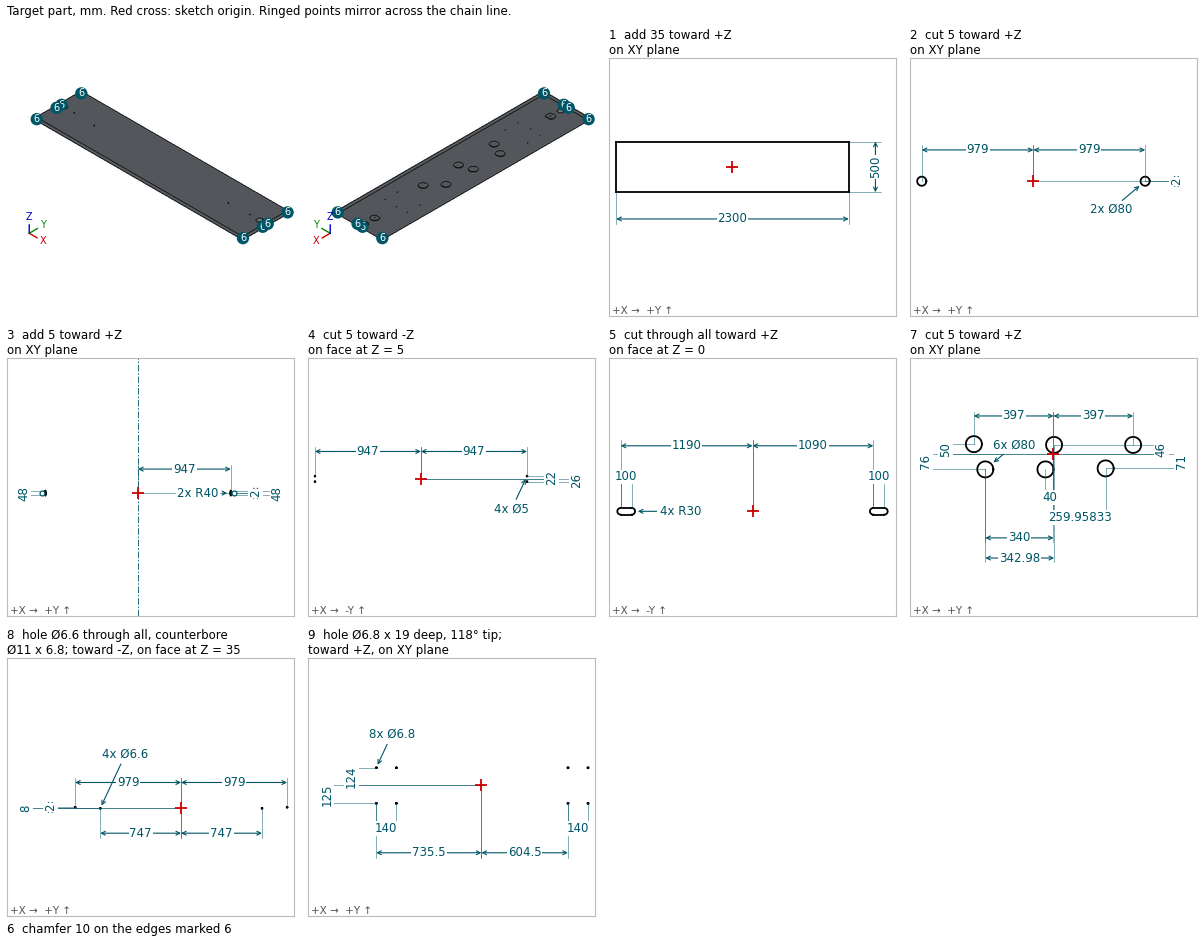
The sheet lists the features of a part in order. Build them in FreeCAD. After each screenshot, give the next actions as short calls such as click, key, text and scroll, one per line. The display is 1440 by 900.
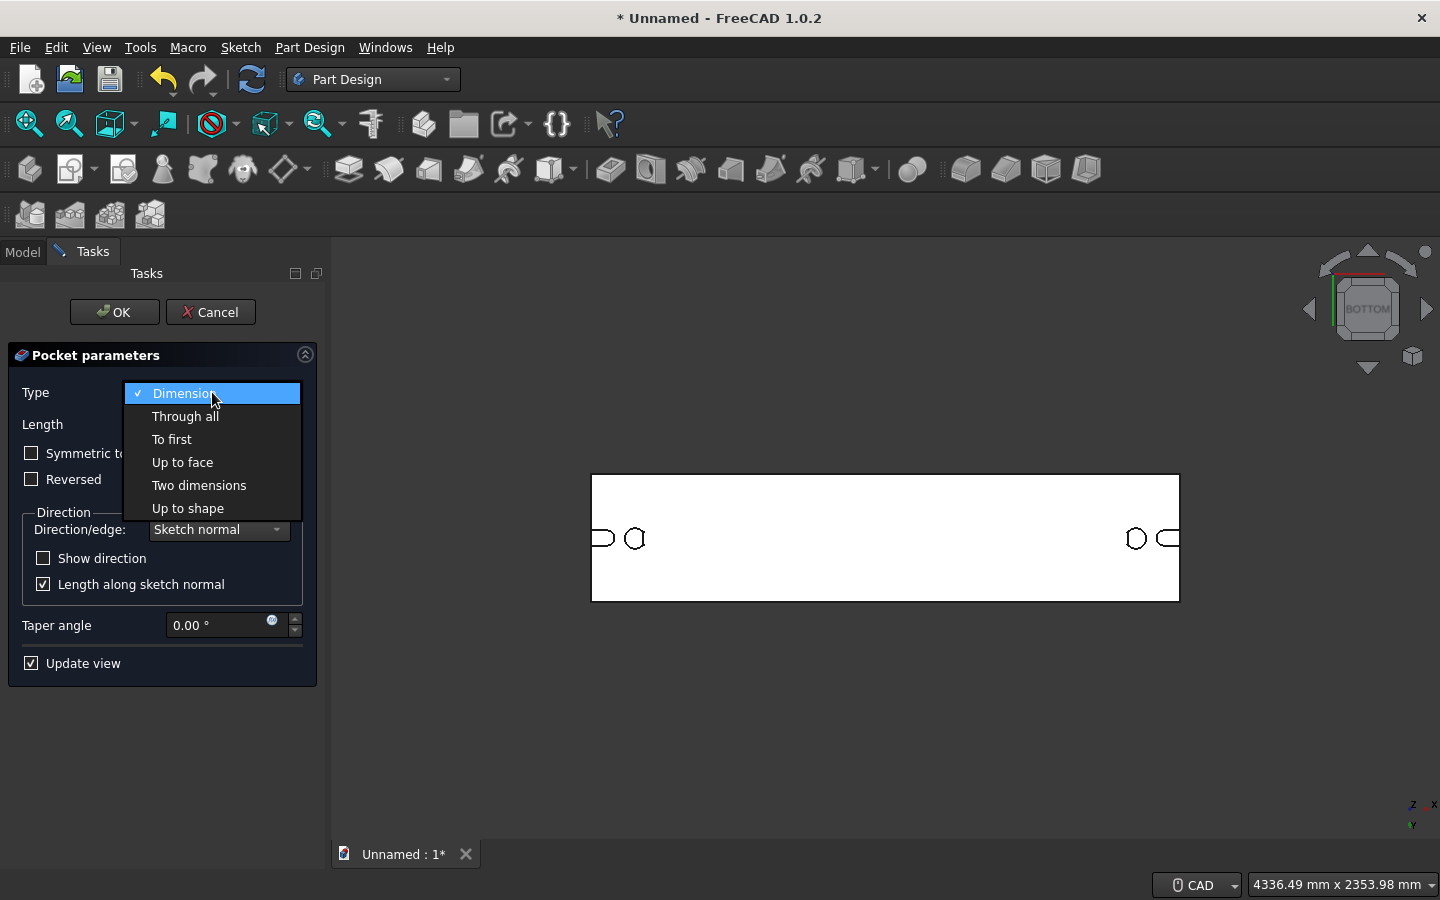
click(212, 416)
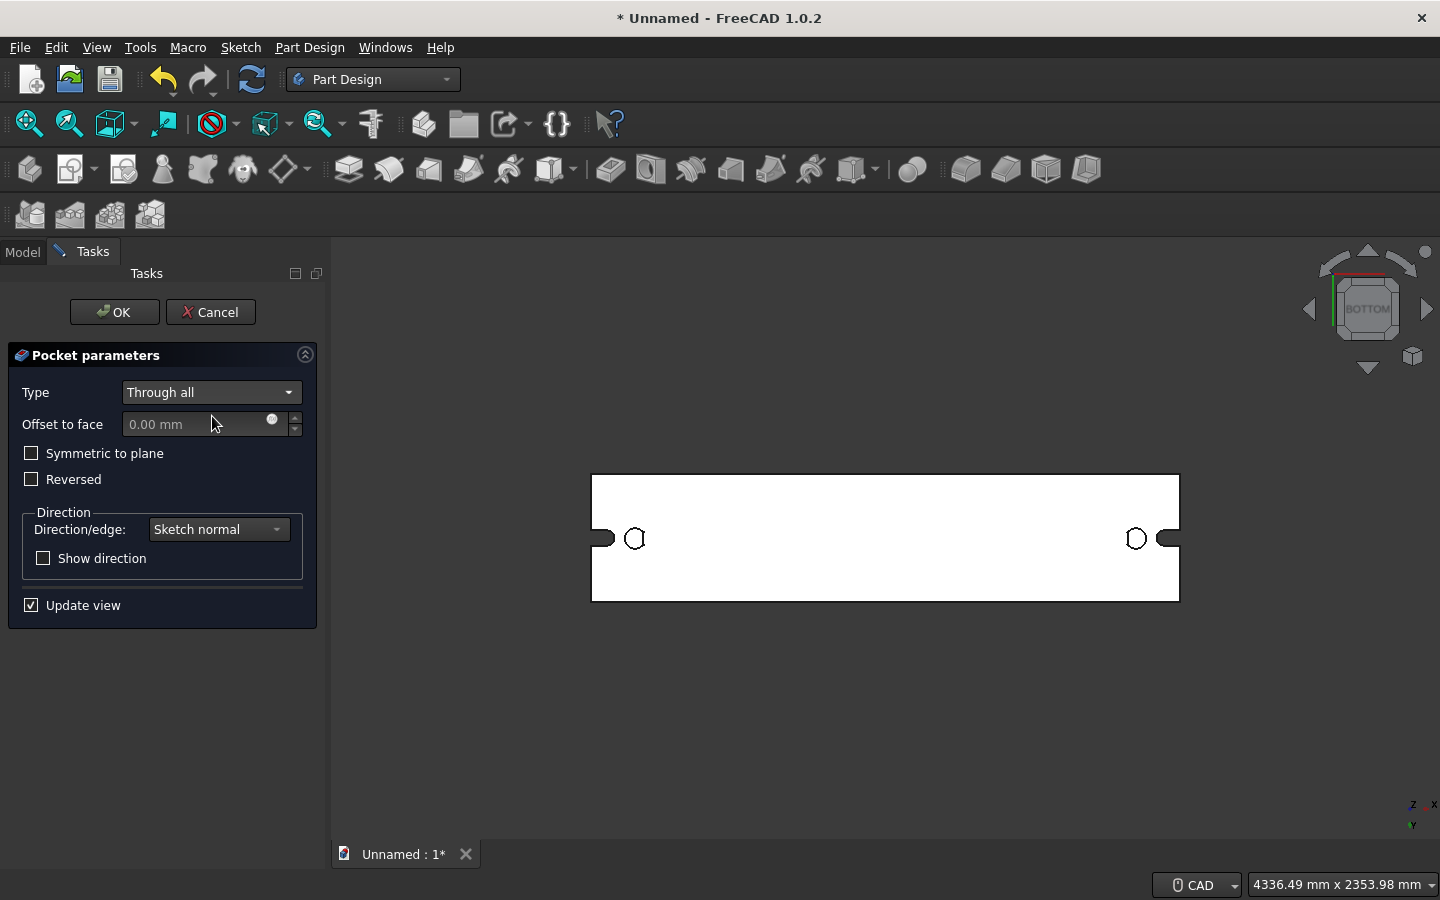
click(115, 312)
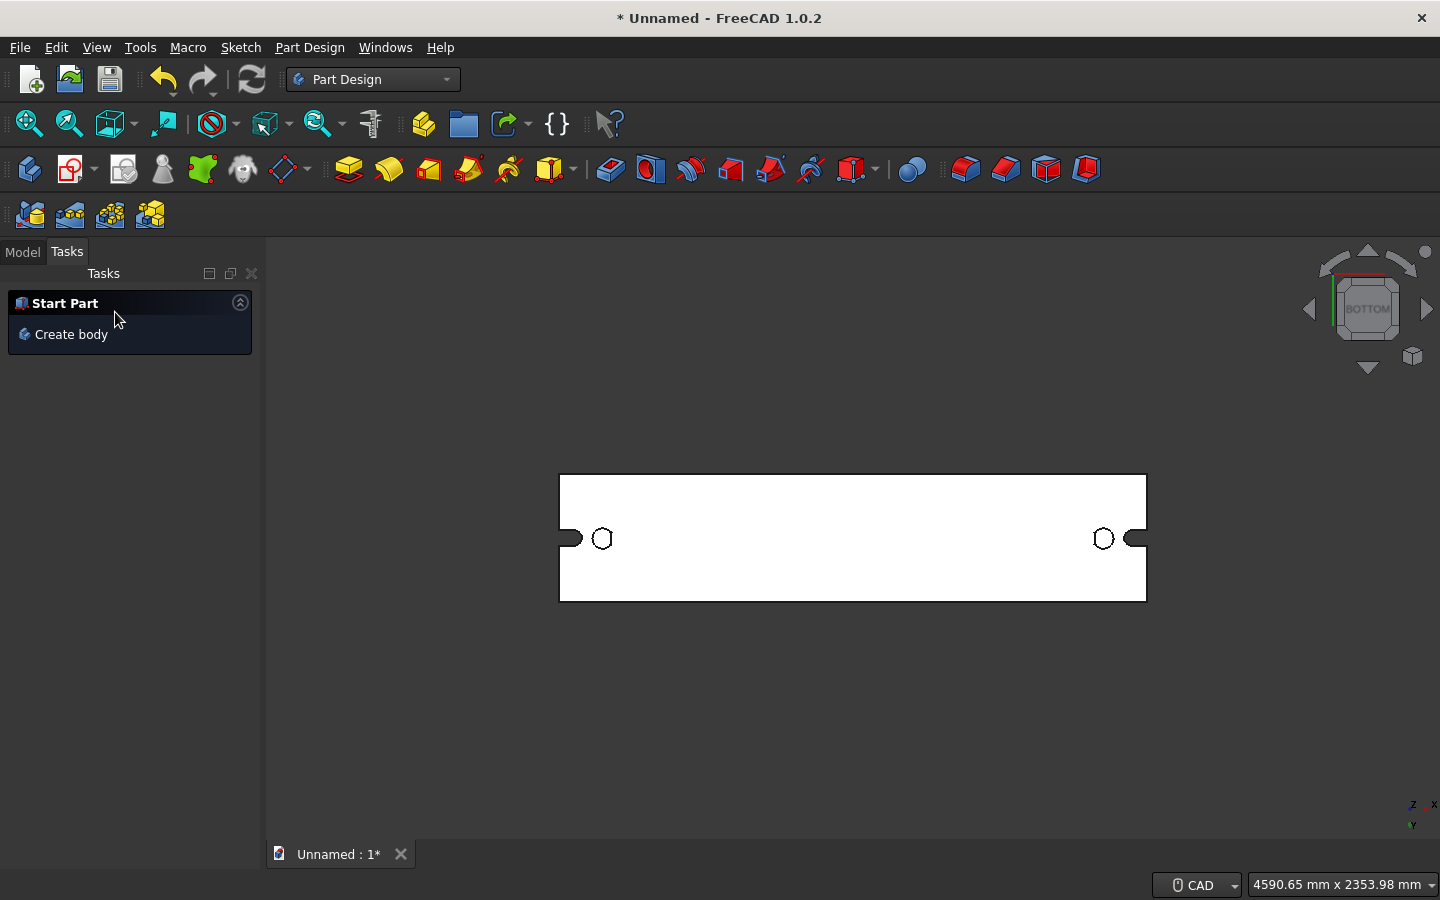
scroll(559, 545, up, 8)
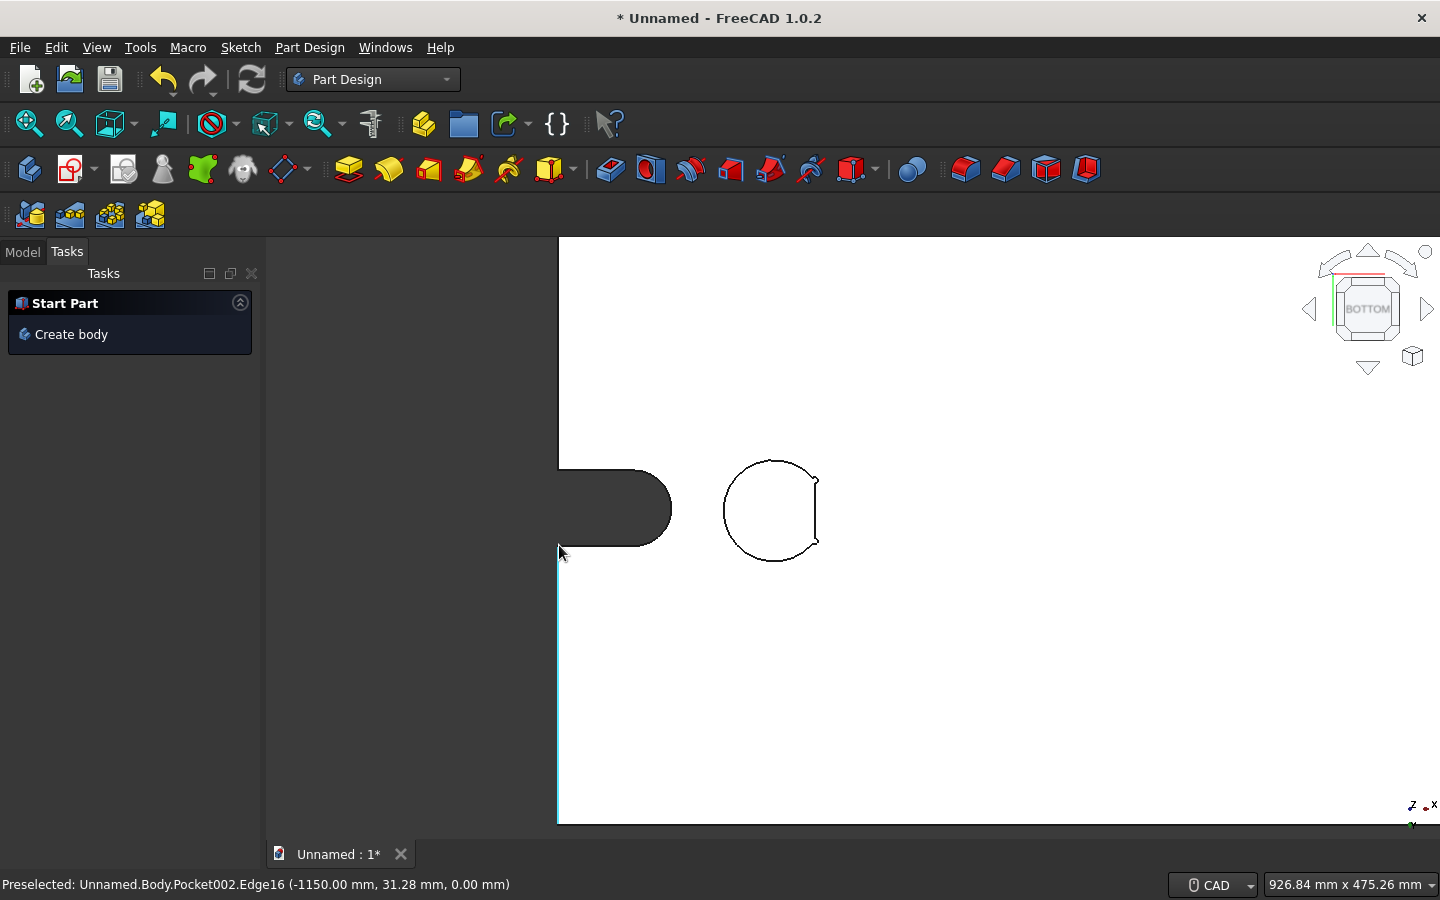
click(30, 124)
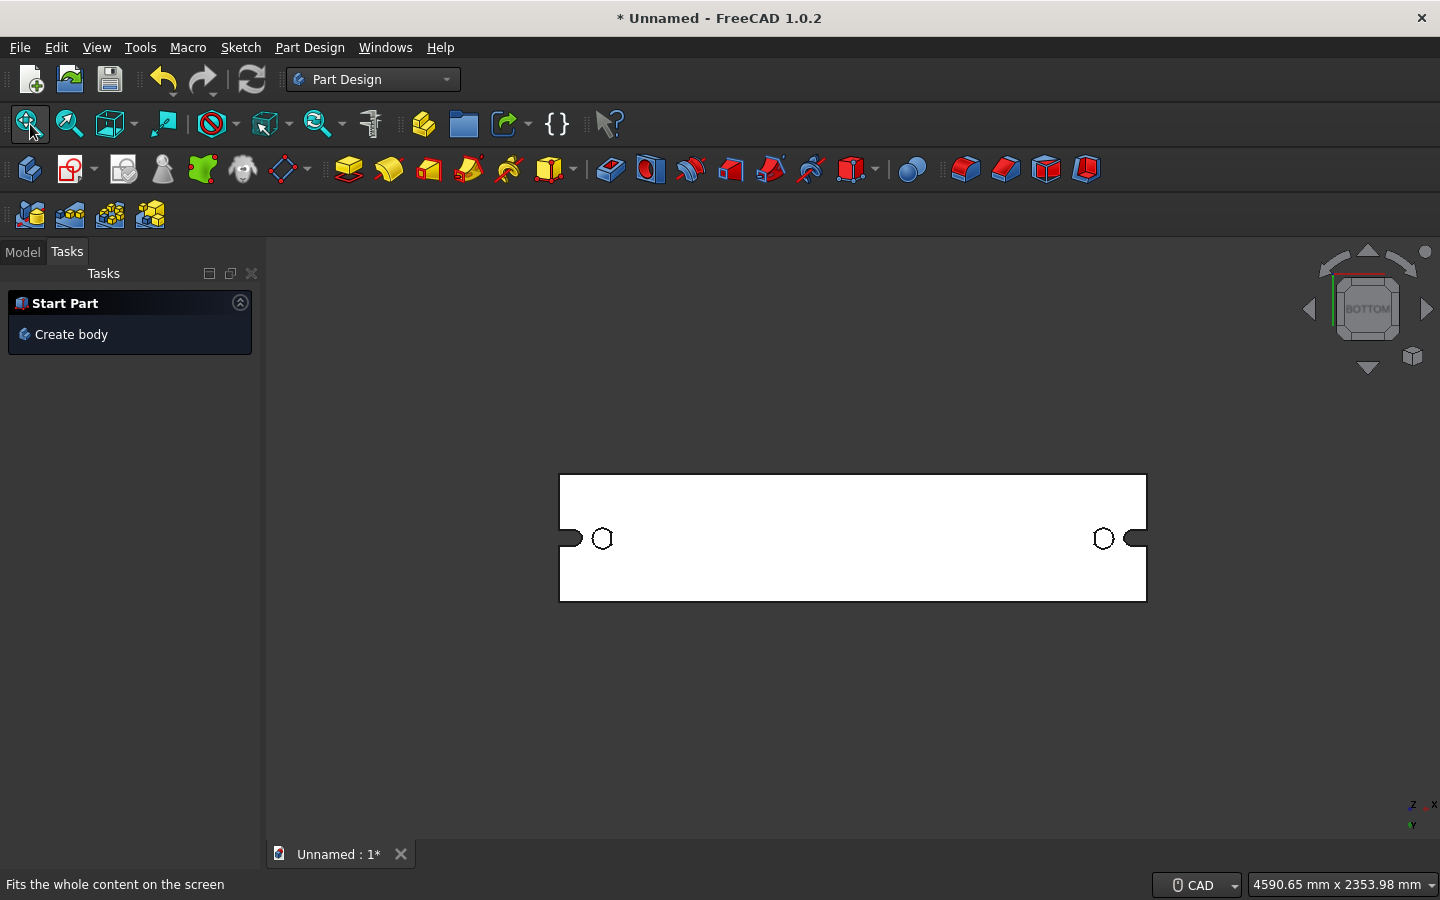
key(0)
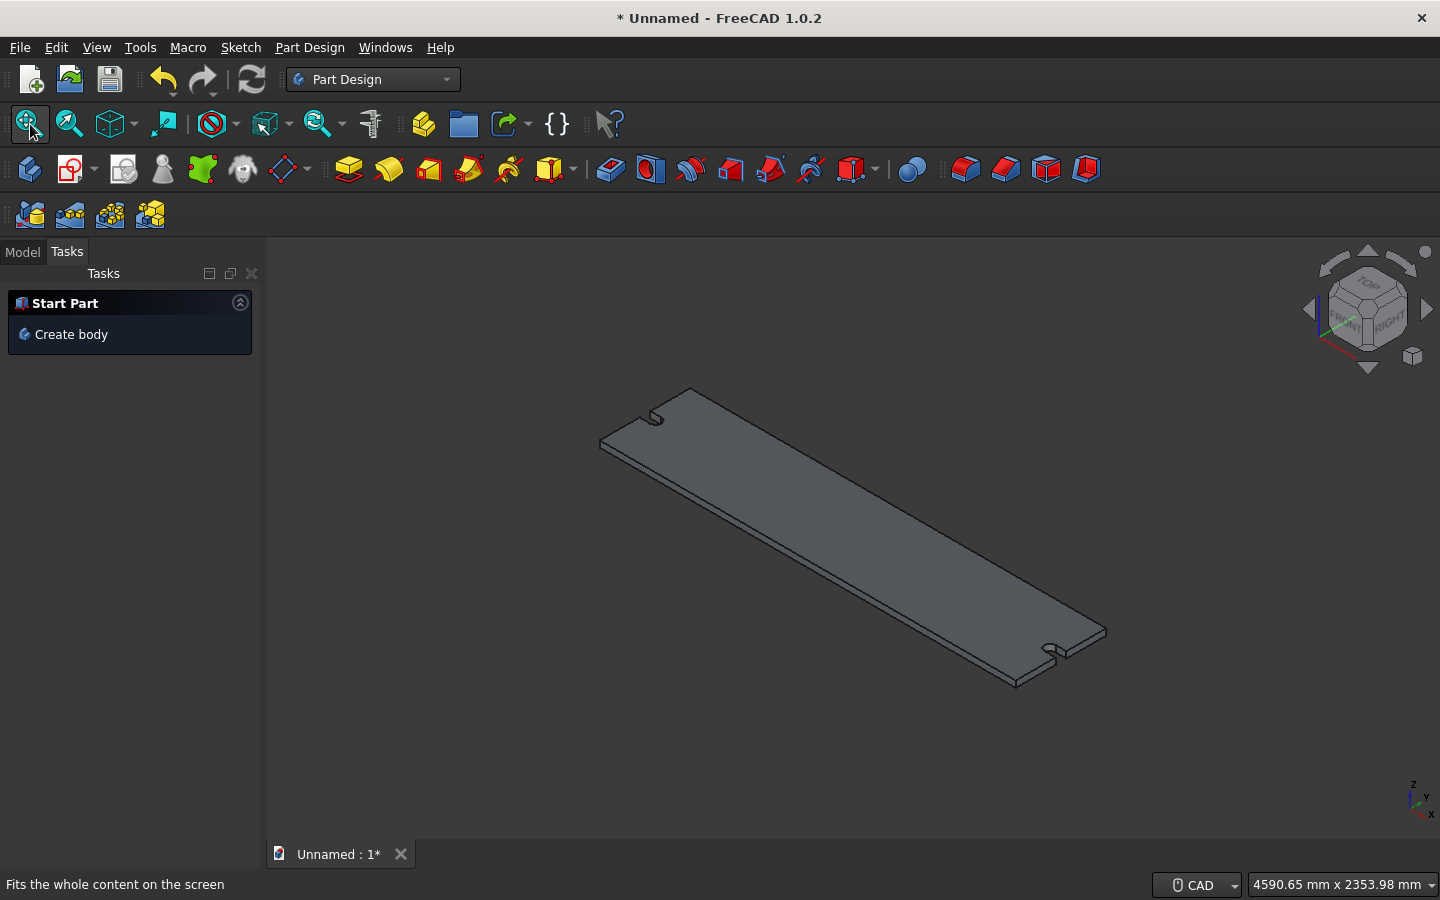
scroll(650, 414, up, 8)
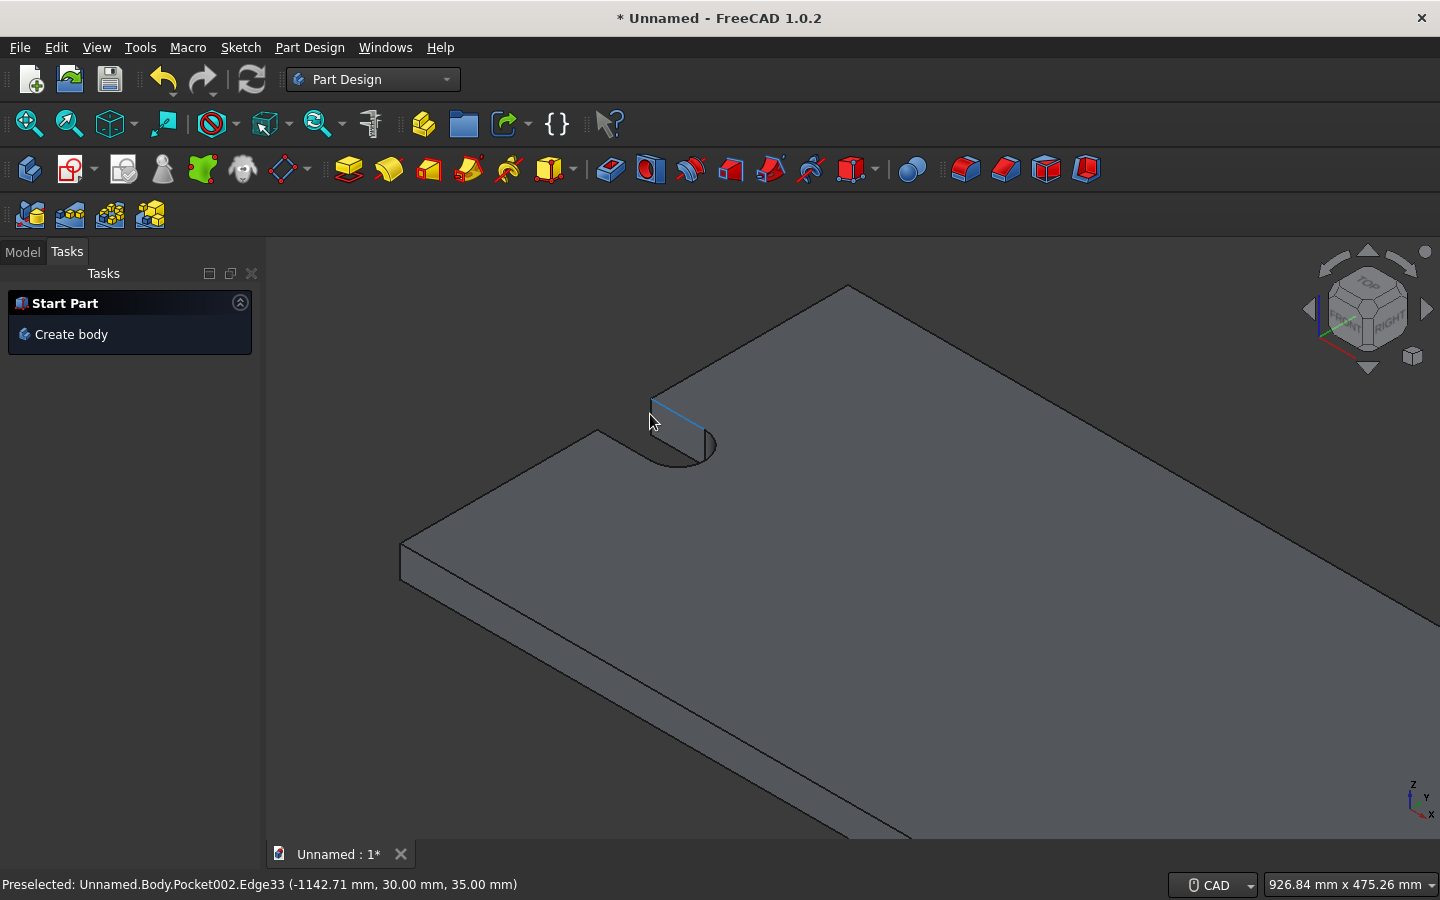
key(v)
key(f)